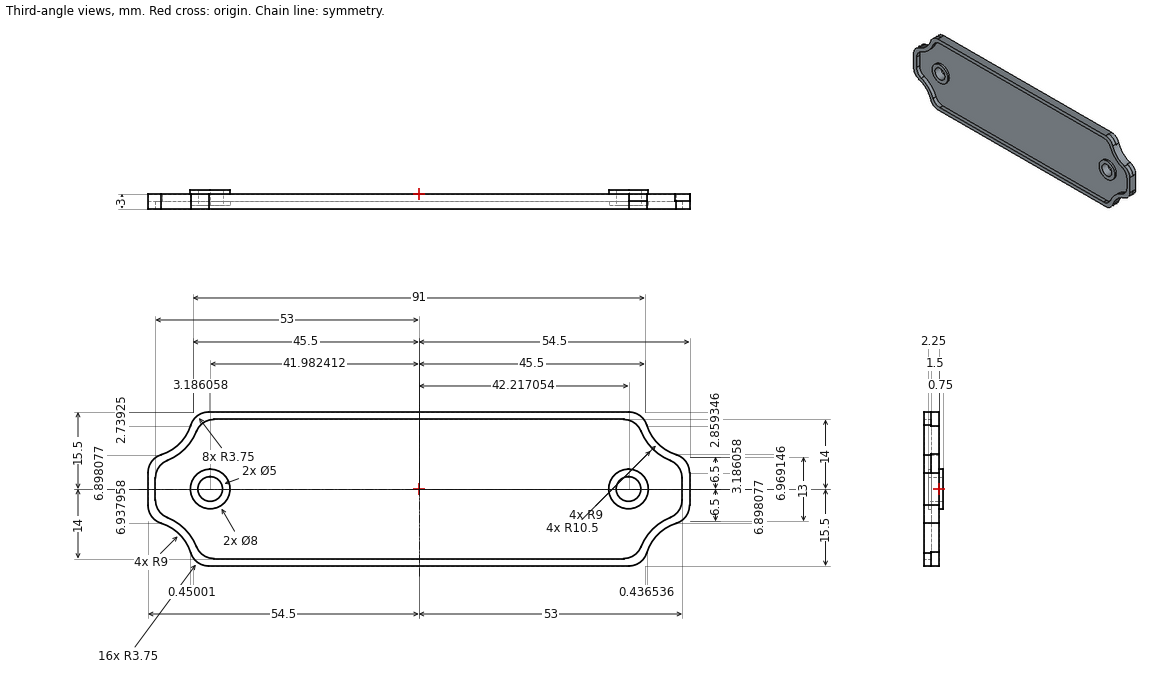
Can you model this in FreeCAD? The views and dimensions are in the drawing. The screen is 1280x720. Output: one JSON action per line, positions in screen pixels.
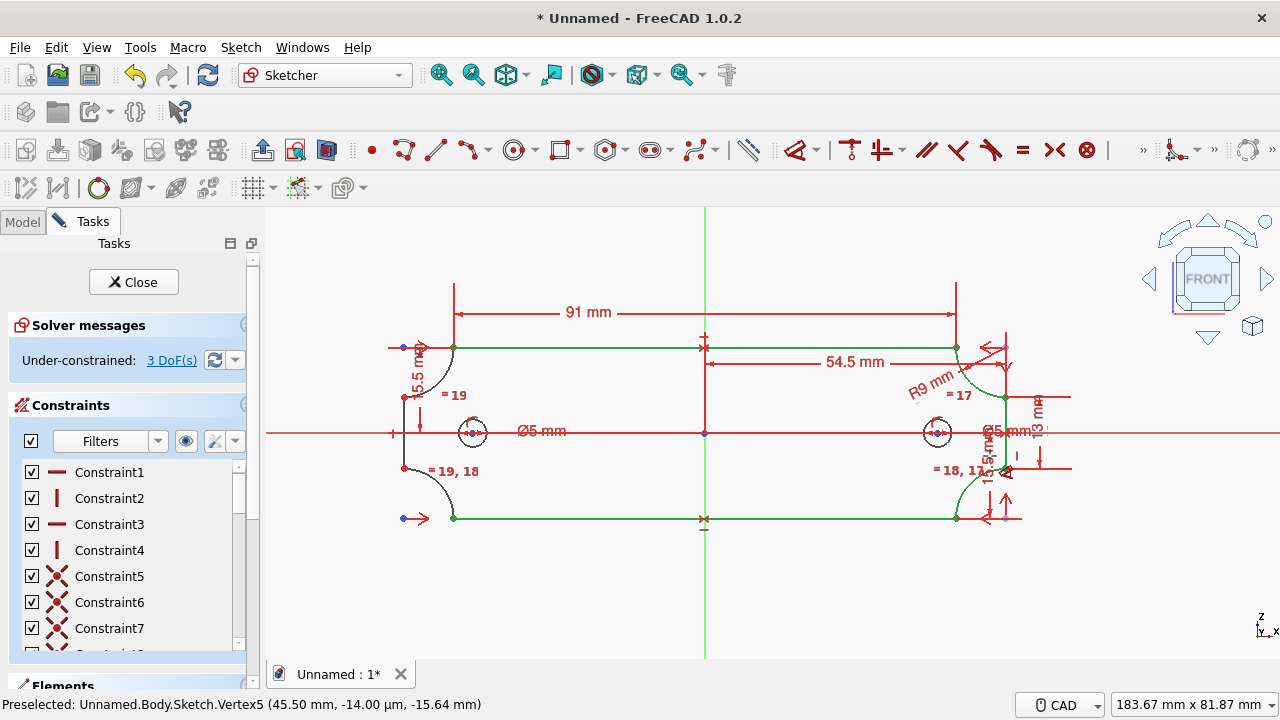
{"action": "left_click", "coordinate": [404, 469]}
{"action": "left_click", "coordinate": [555, 503]}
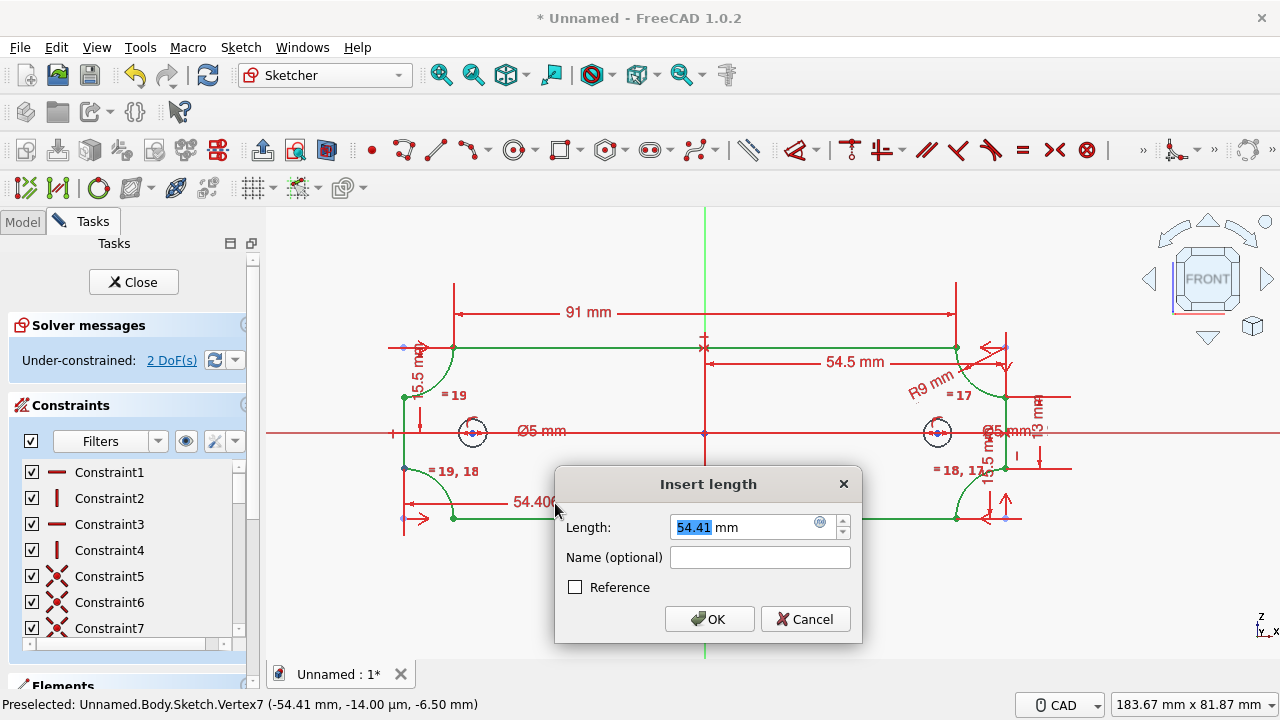
{"action": "type", "text": "54.5"}
{"action": "key", "text": "Return"}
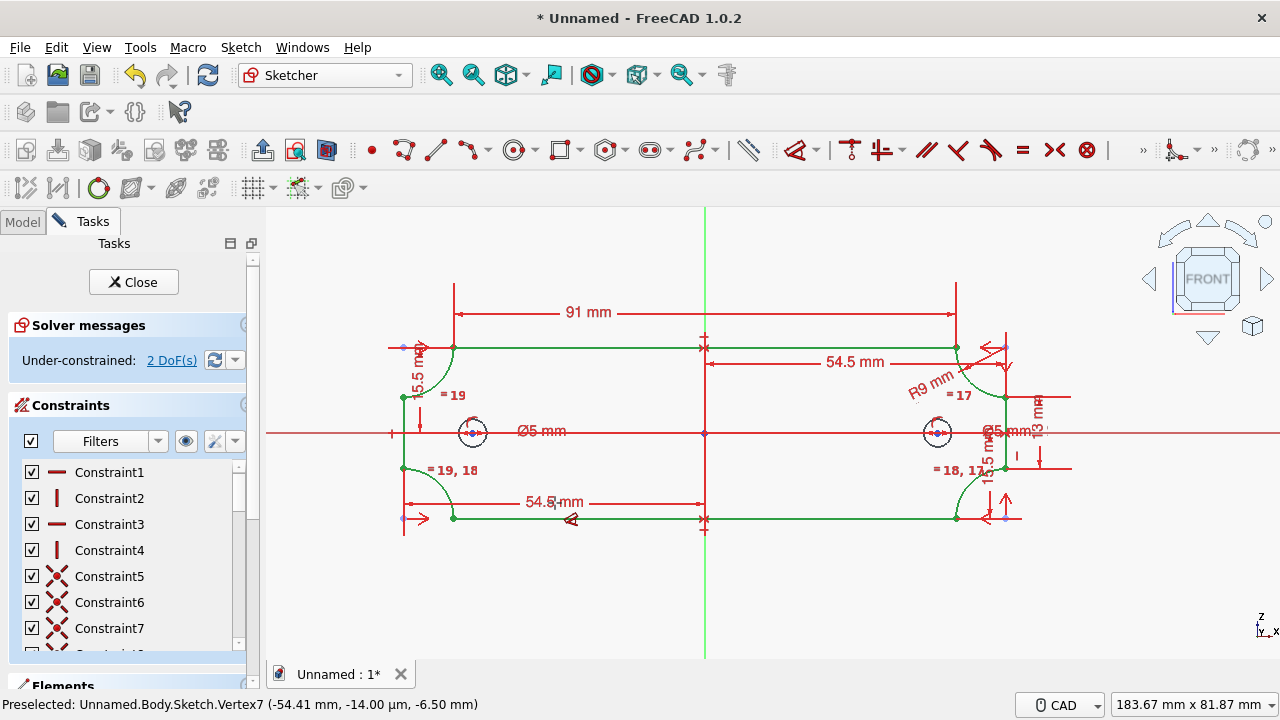
{"action": "left_click", "coordinate": [473, 433]}
{"action": "left_click", "coordinate": [589, 467]}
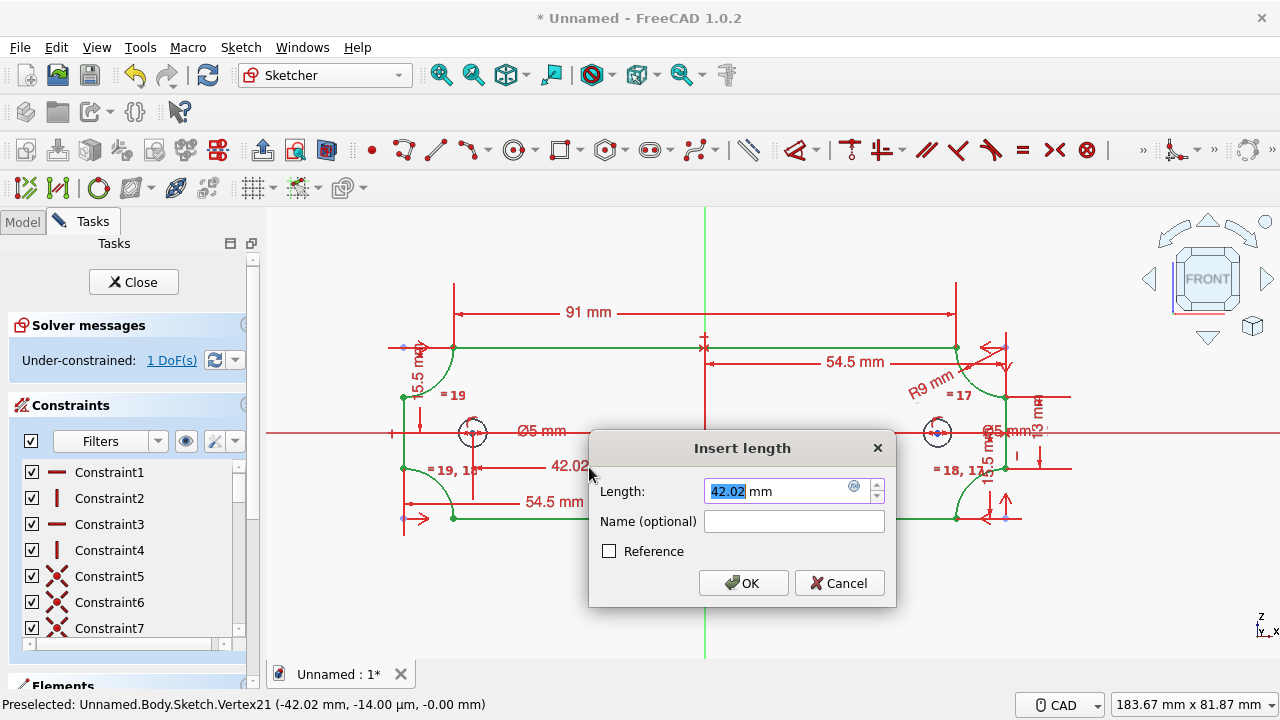
{"action": "type", "text": "41.982412"}
{"action": "key", "text": "Return"}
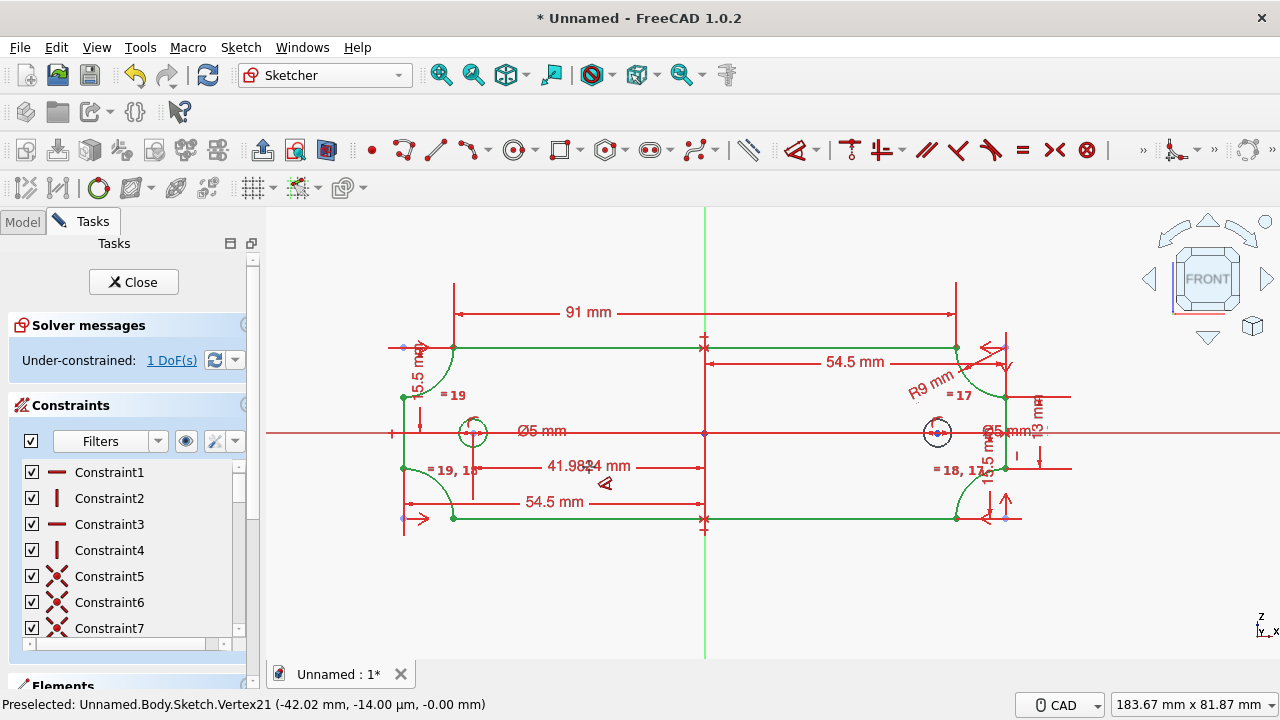
{"action": "left_click", "coordinate": [938, 433]}
{"action": "left_click", "coordinate": [821, 467]}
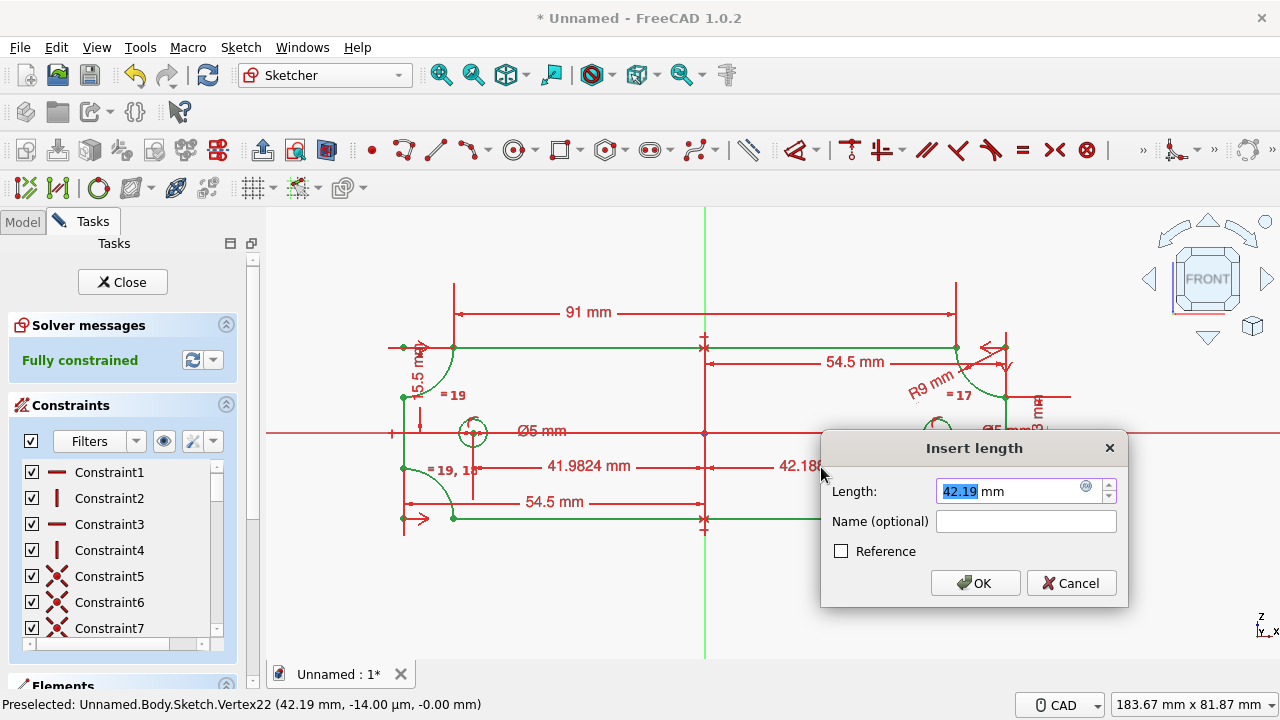
{"action": "type", "text": "42.217054"}
{"action": "key", "text": "Return"}
{"action": "key", "text": "Escape"}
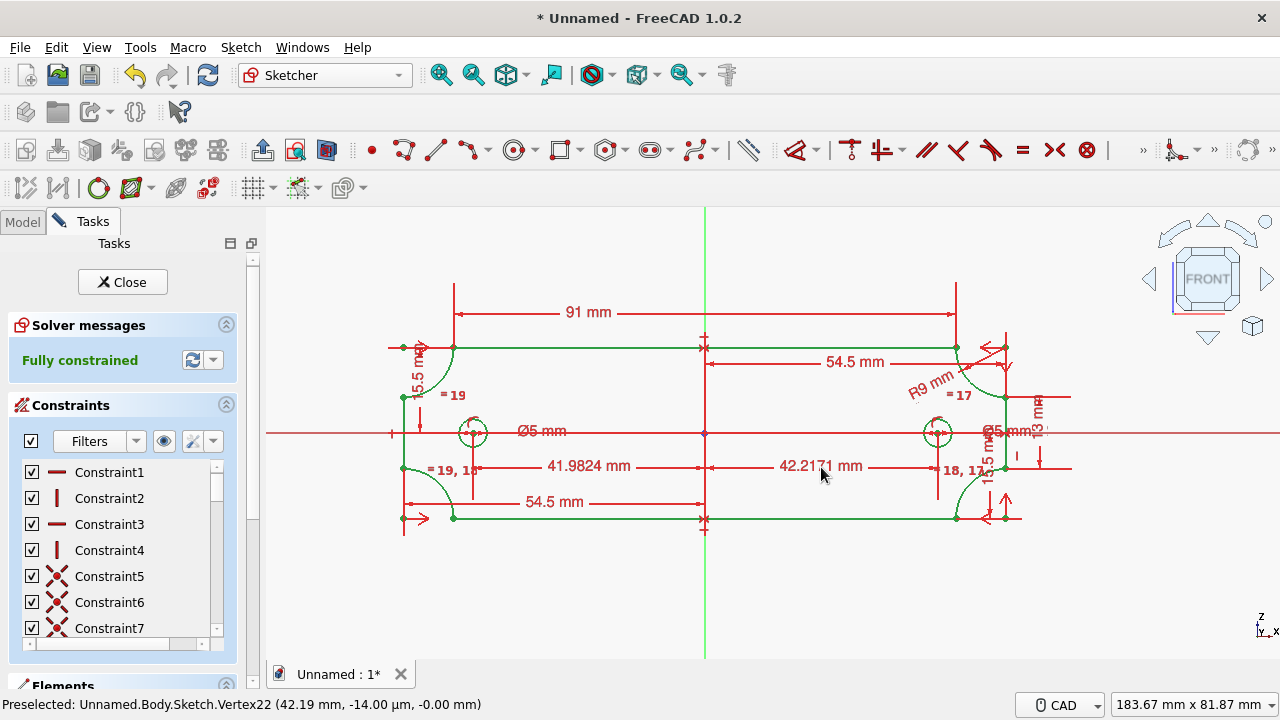
{"action": "left_click", "coordinate": [123, 282]}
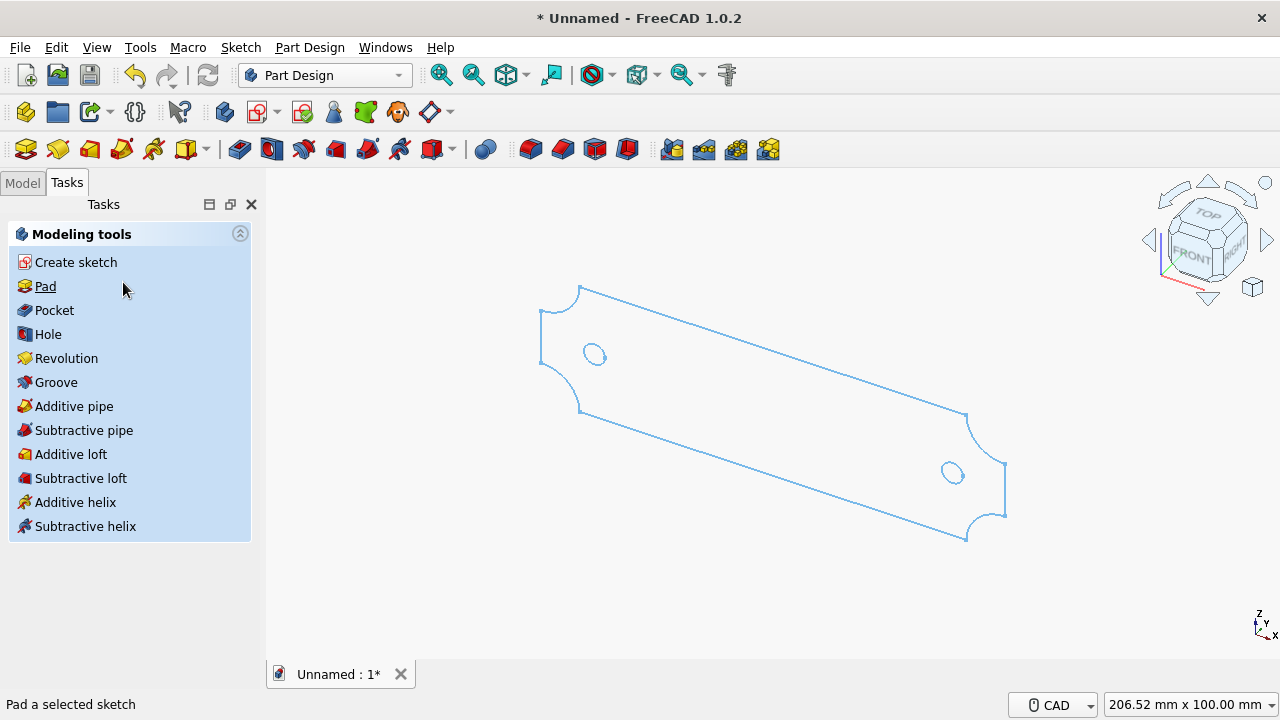
{"action": "left_click", "coordinate": [26, 150]}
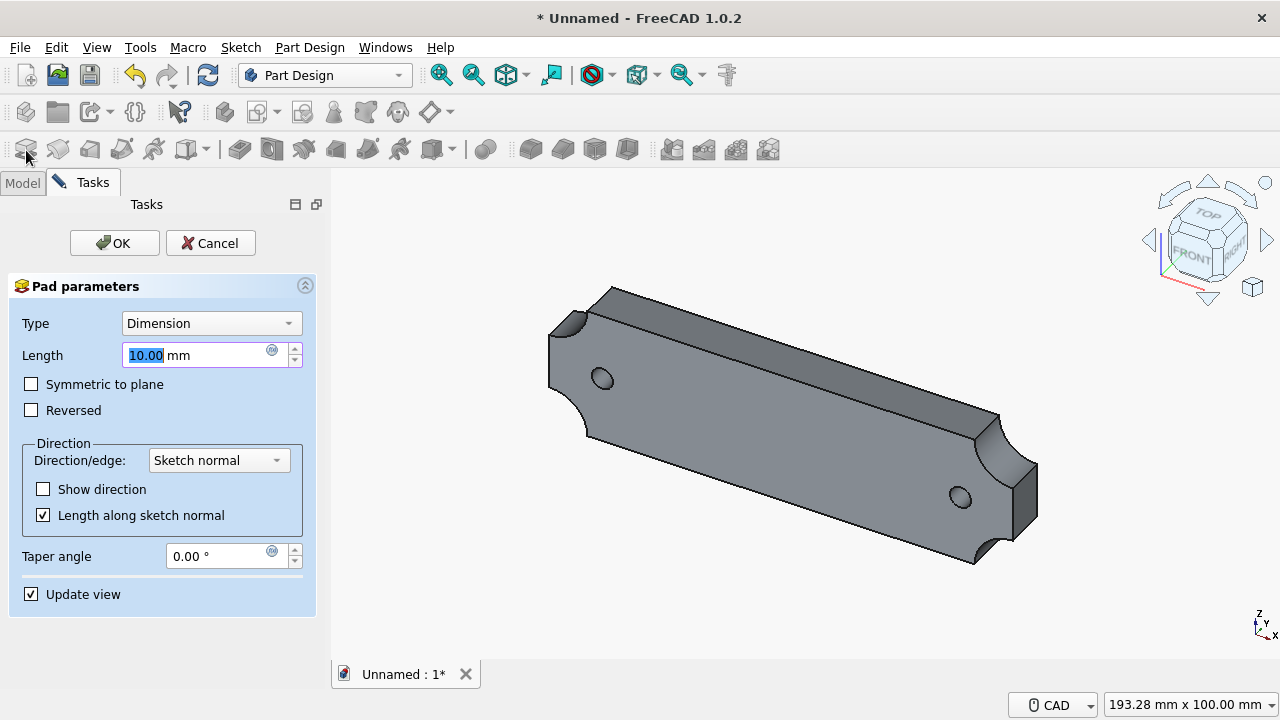
{"action": "type", "text": "1.5"}
{"action": "key", "text": "Tab"}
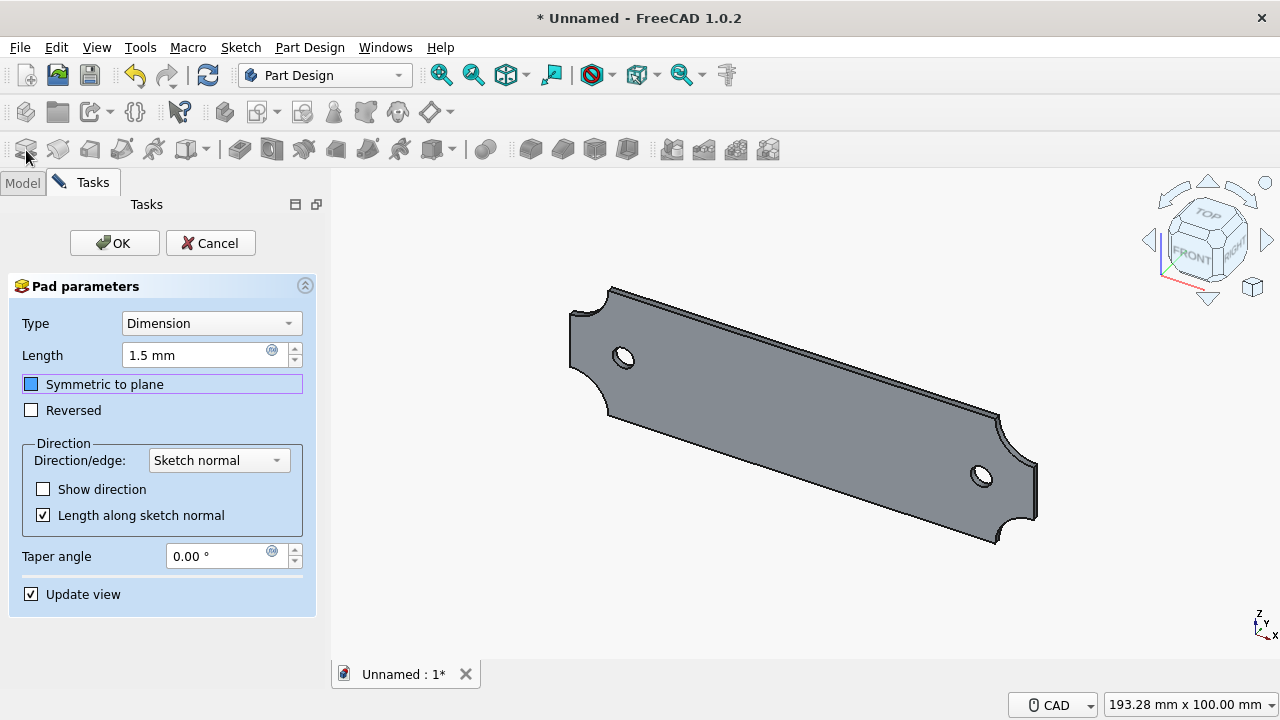
{"action": "left_click", "coordinate": [115, 243]}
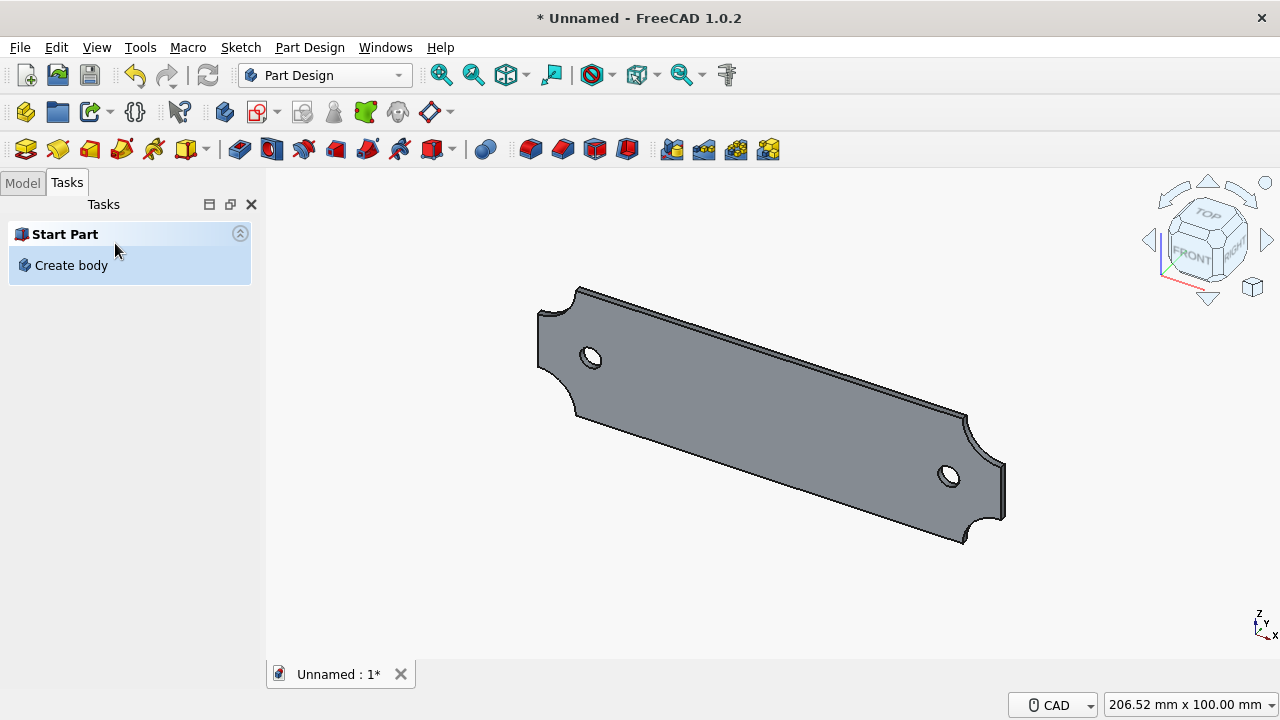
{"action": "key", "text": "4"}